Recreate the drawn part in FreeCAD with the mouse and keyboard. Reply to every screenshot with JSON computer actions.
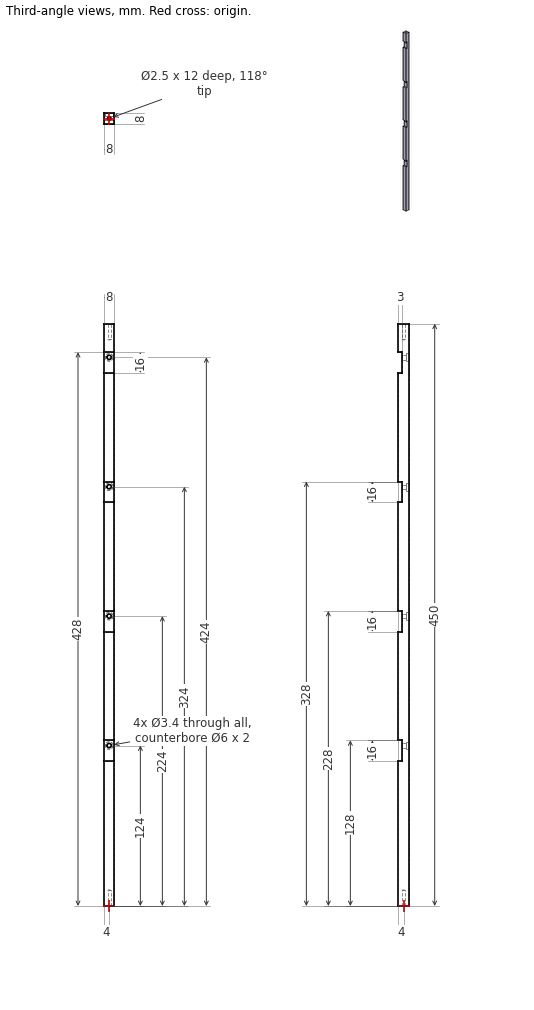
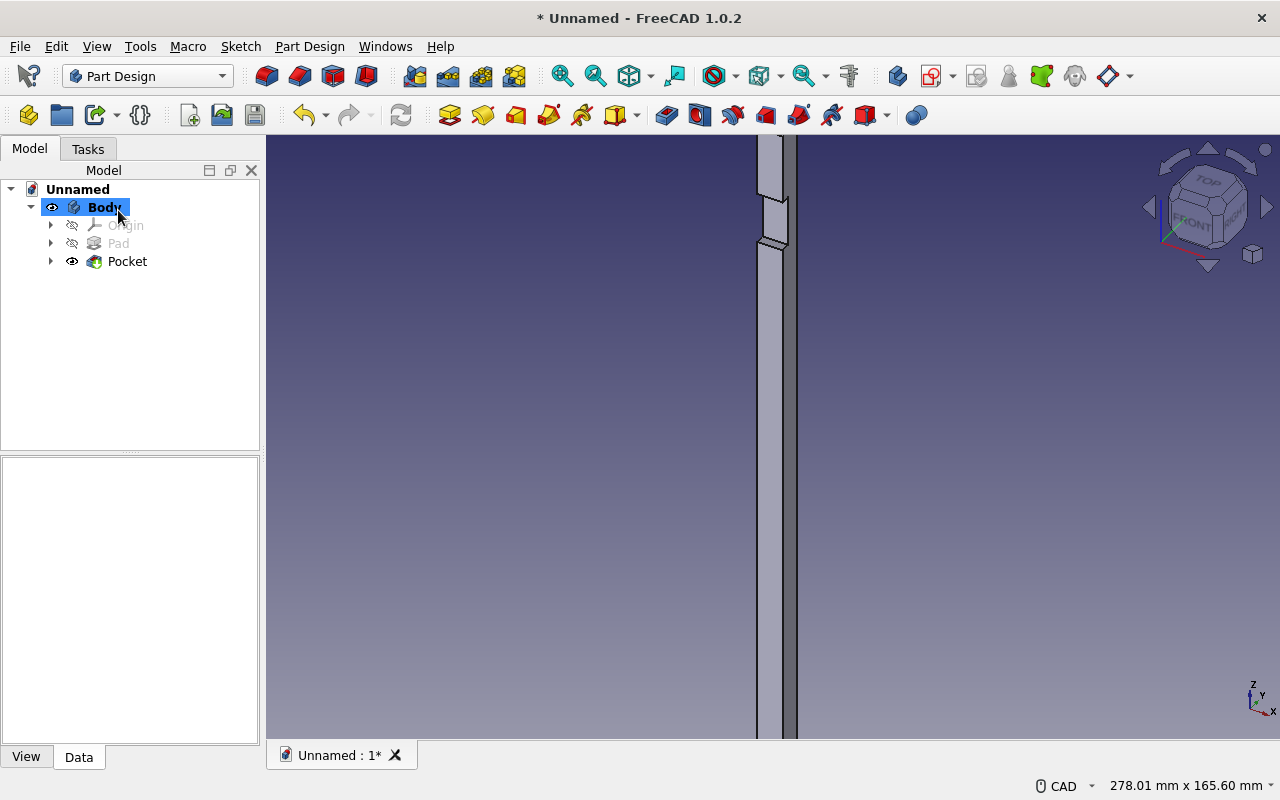
{"action": "key", "text": "v f"}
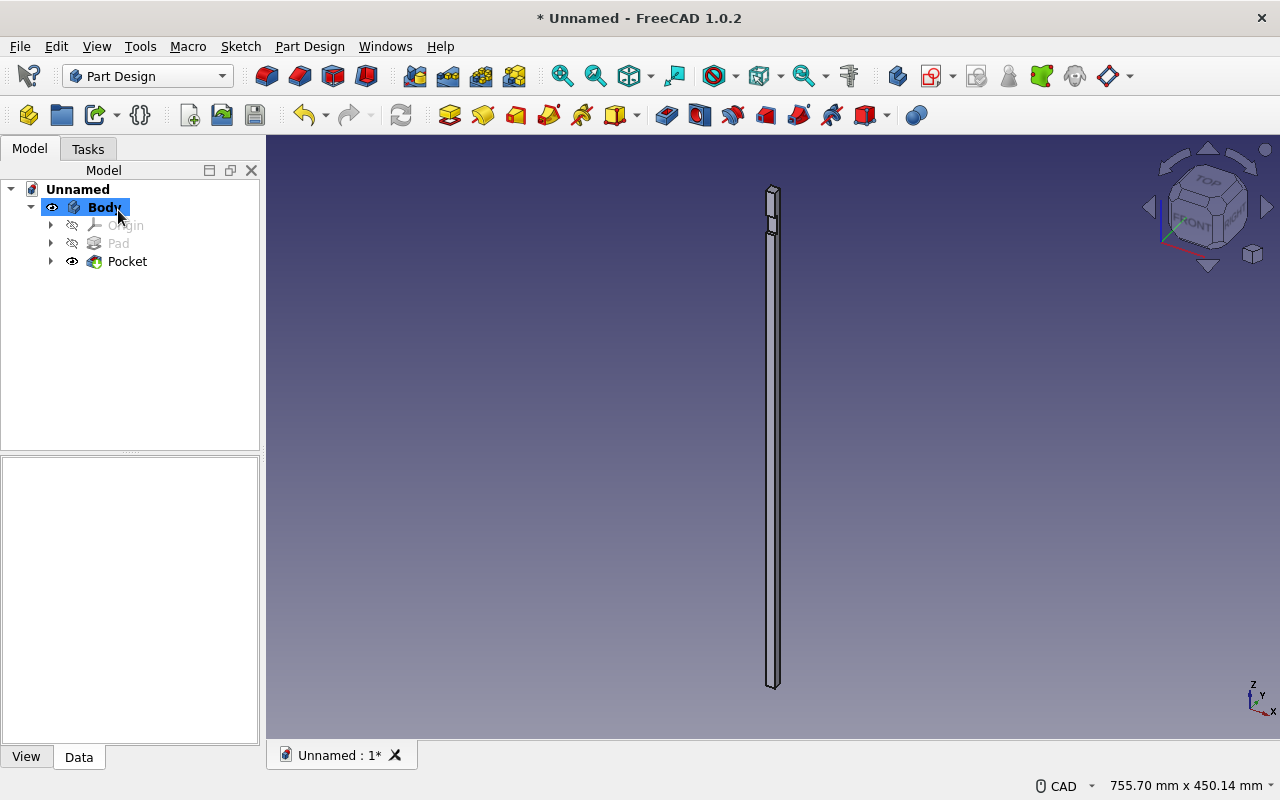
{"action": "key", "text": "5"}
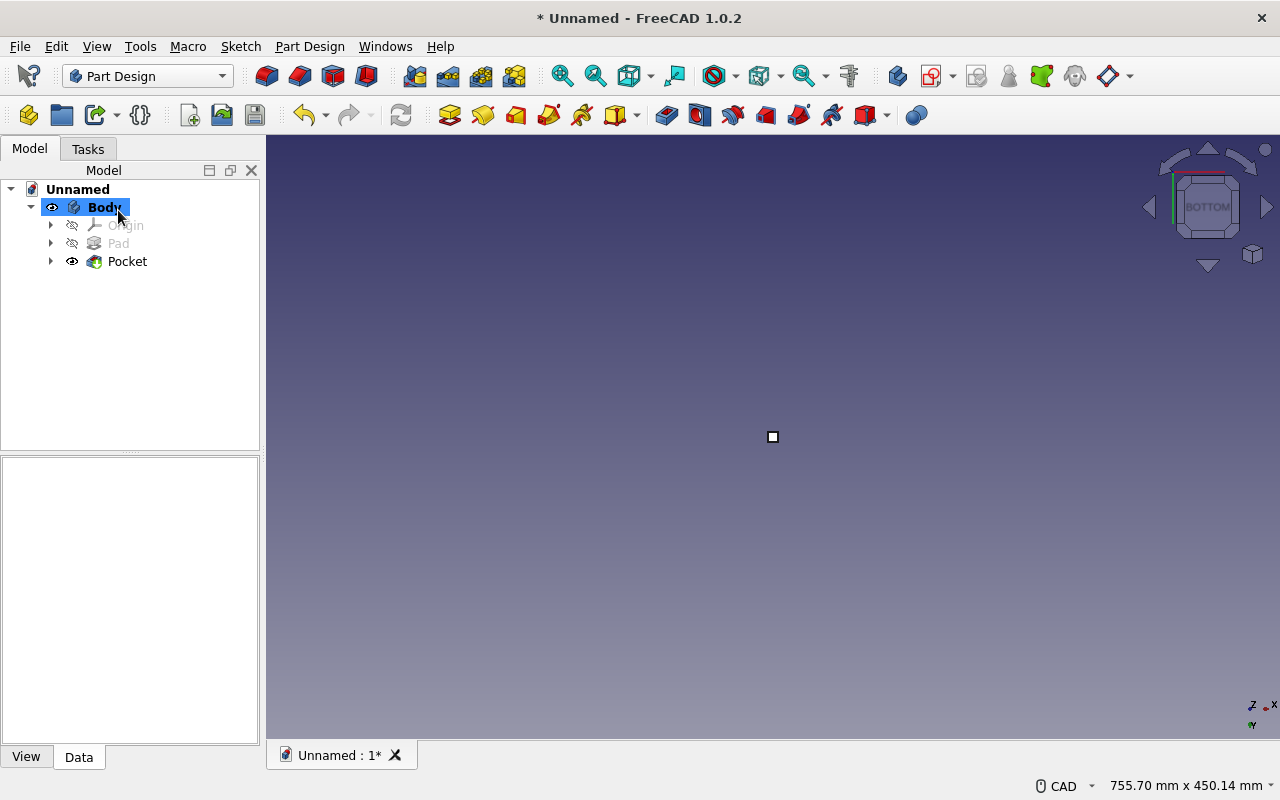
{"action": "key", "text": "v f"}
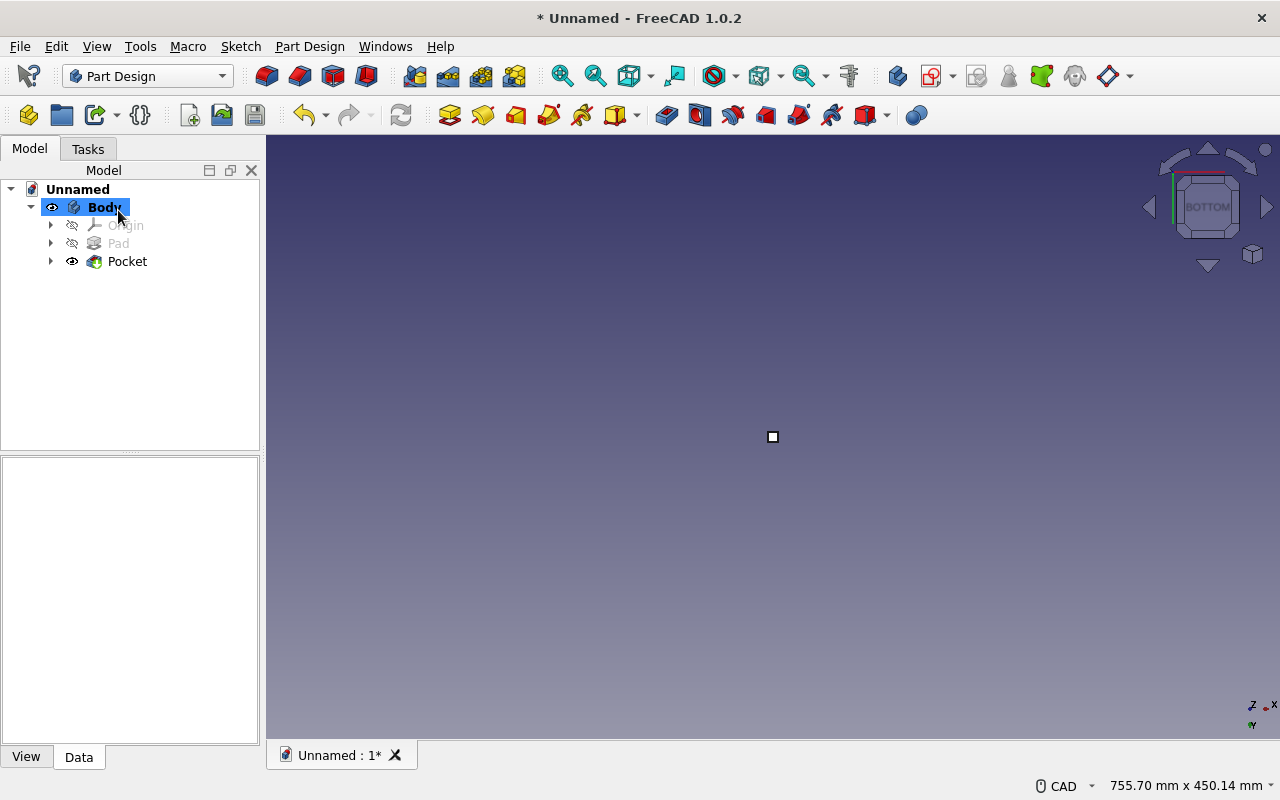
{"action": "scroll", "coordinate": [773, 436], "scroll_direction": "up", "scroll_amount": 5}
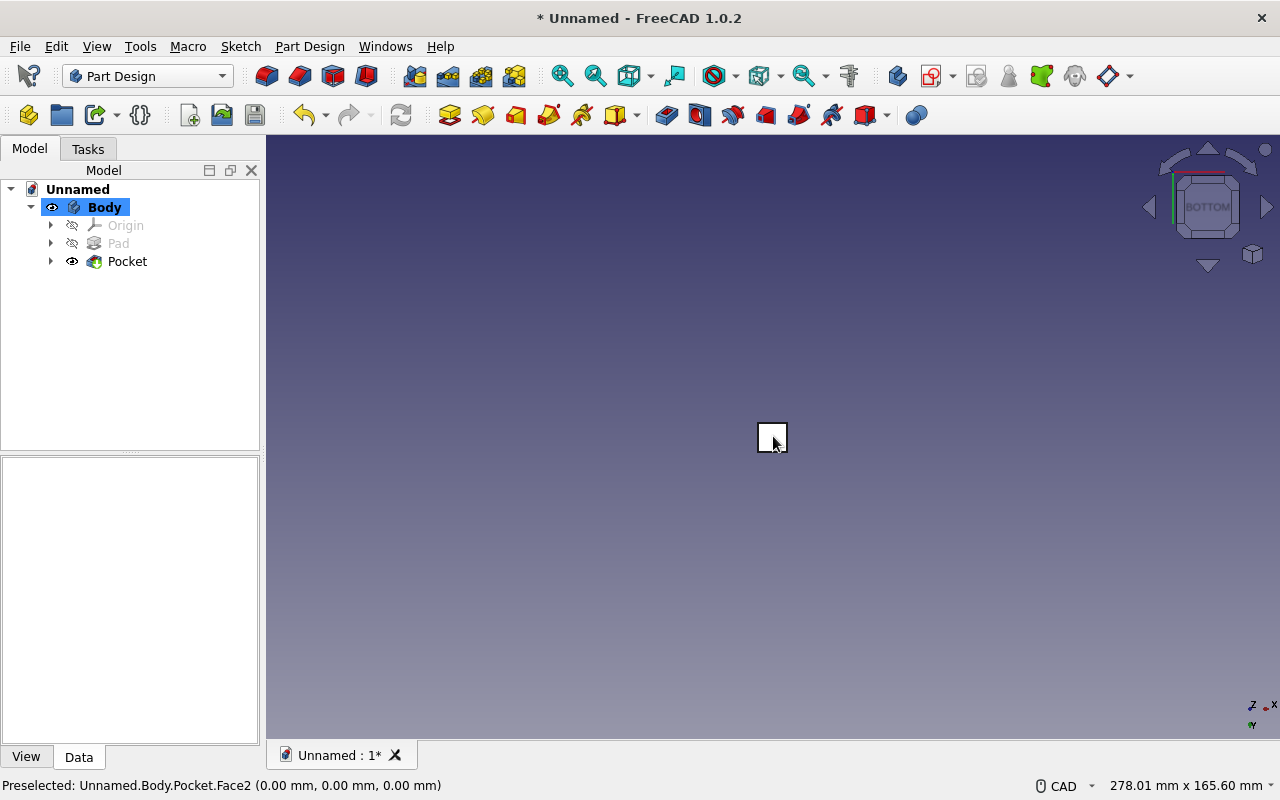
{"action": "left_click", "coordinate": [772, 437]}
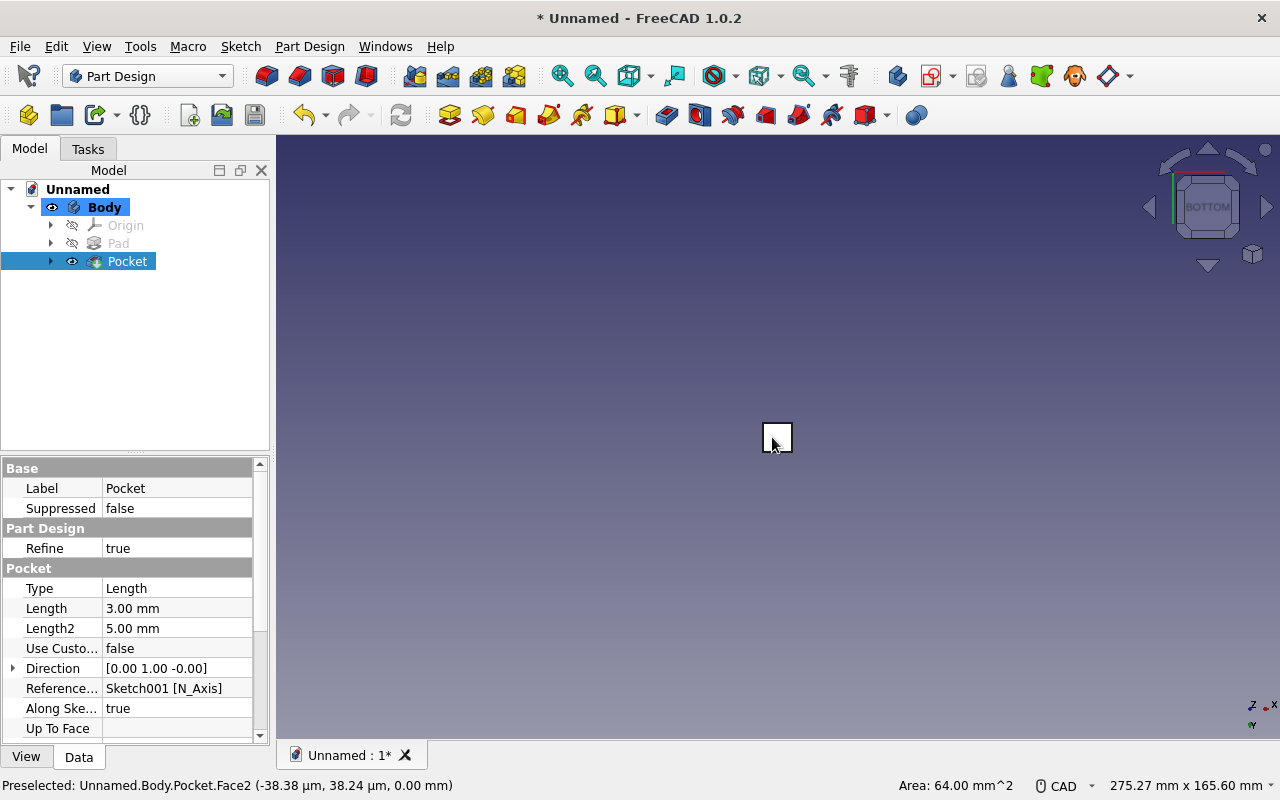
{"action": "left_click", "coordinate": [930, 76]}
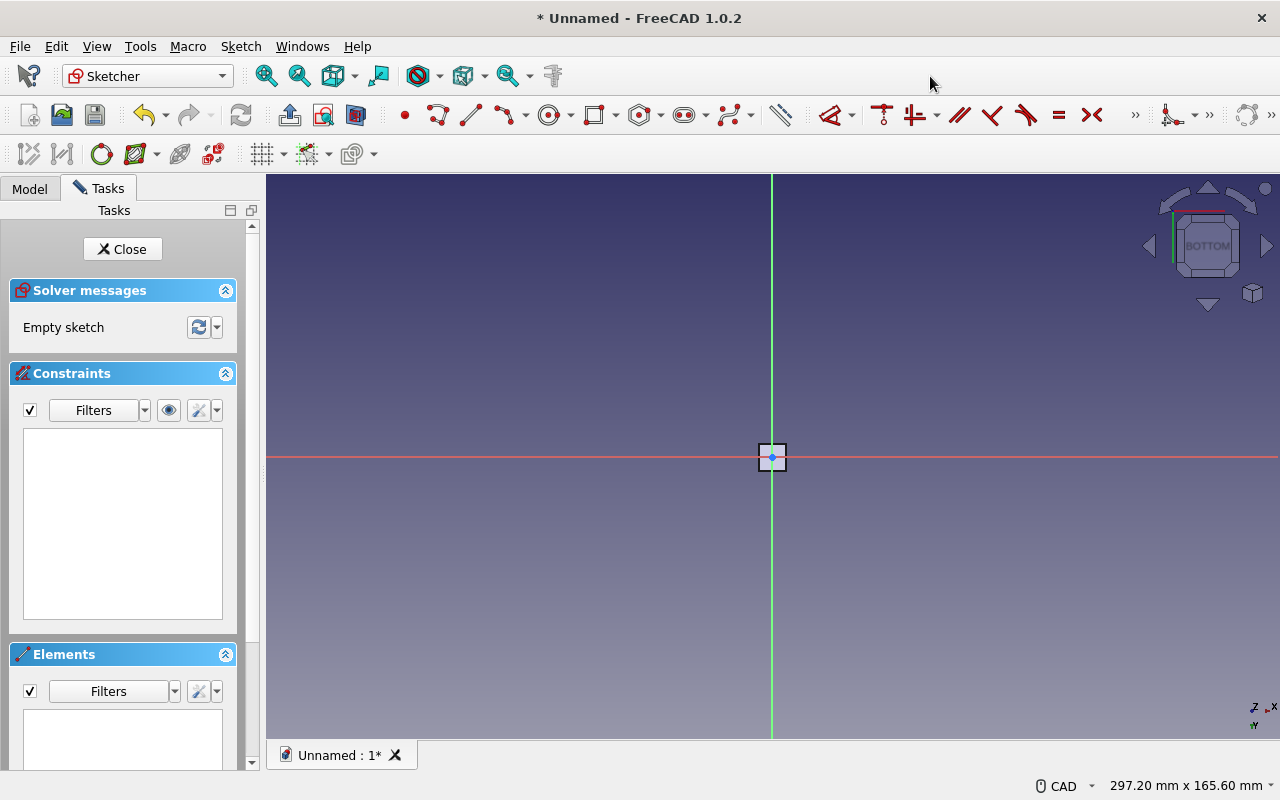
{"action": "scroll", "coordinate": [776, 457], "scroll_direction": "up", "scroll_amount": 15}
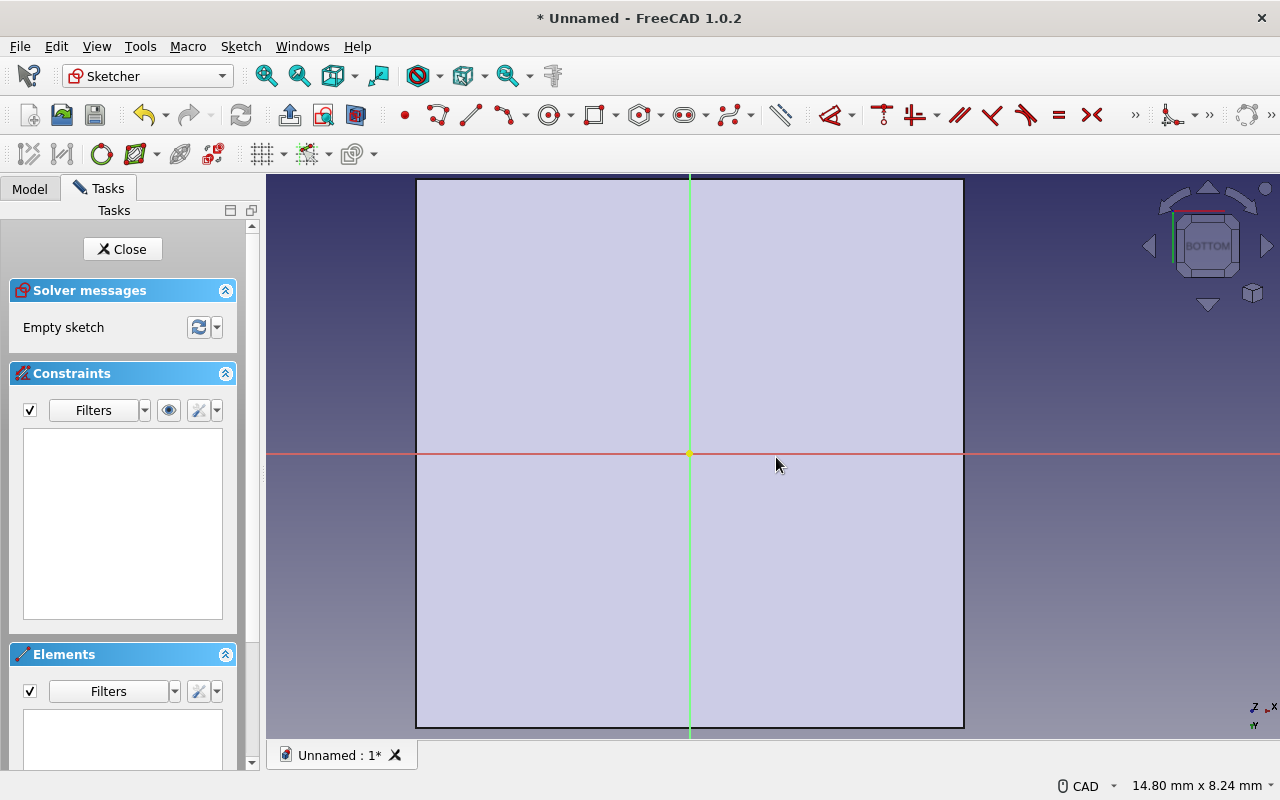
{"action": "scroll", "coordinate": [678, 451], "scroll_direction": "up", "scroll_amount": 4}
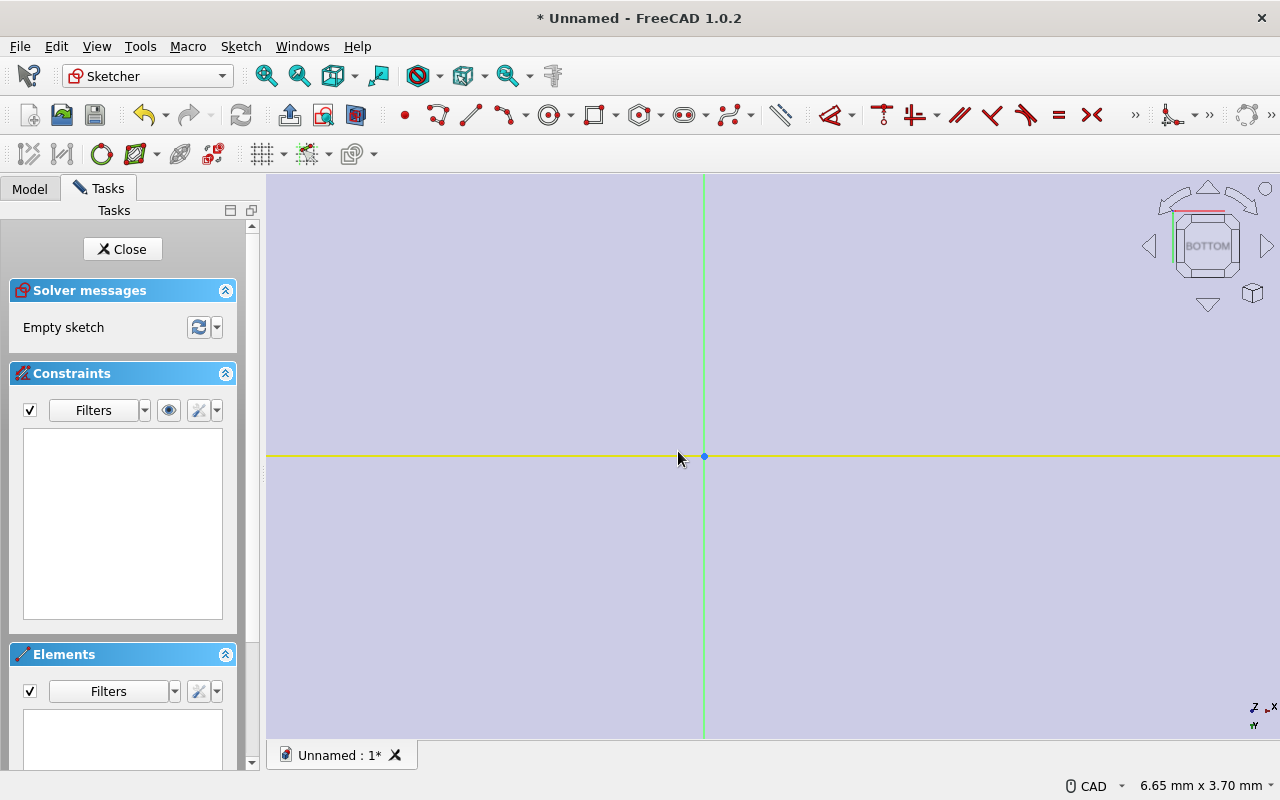
{"action": "left_click", "coordinate": [548, 116]}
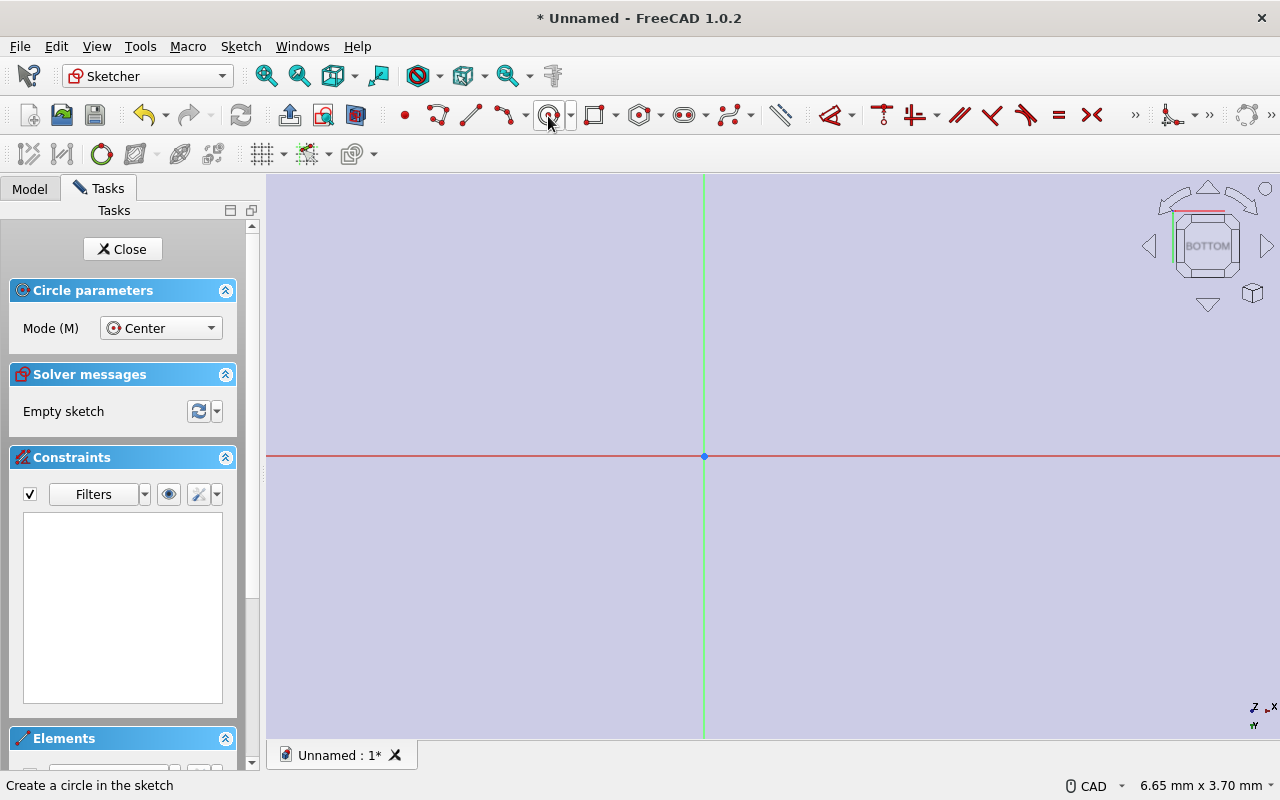
{"action": "left_click", "coordinate": [704, 456]}
{"action": "mouse_move", "coordinate": [839, 321]}